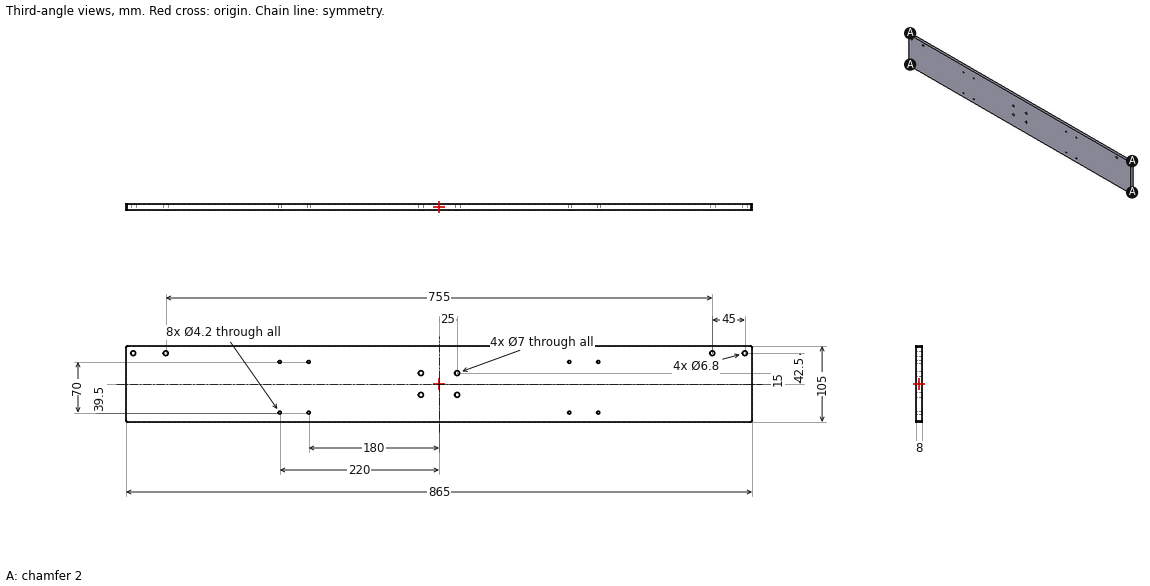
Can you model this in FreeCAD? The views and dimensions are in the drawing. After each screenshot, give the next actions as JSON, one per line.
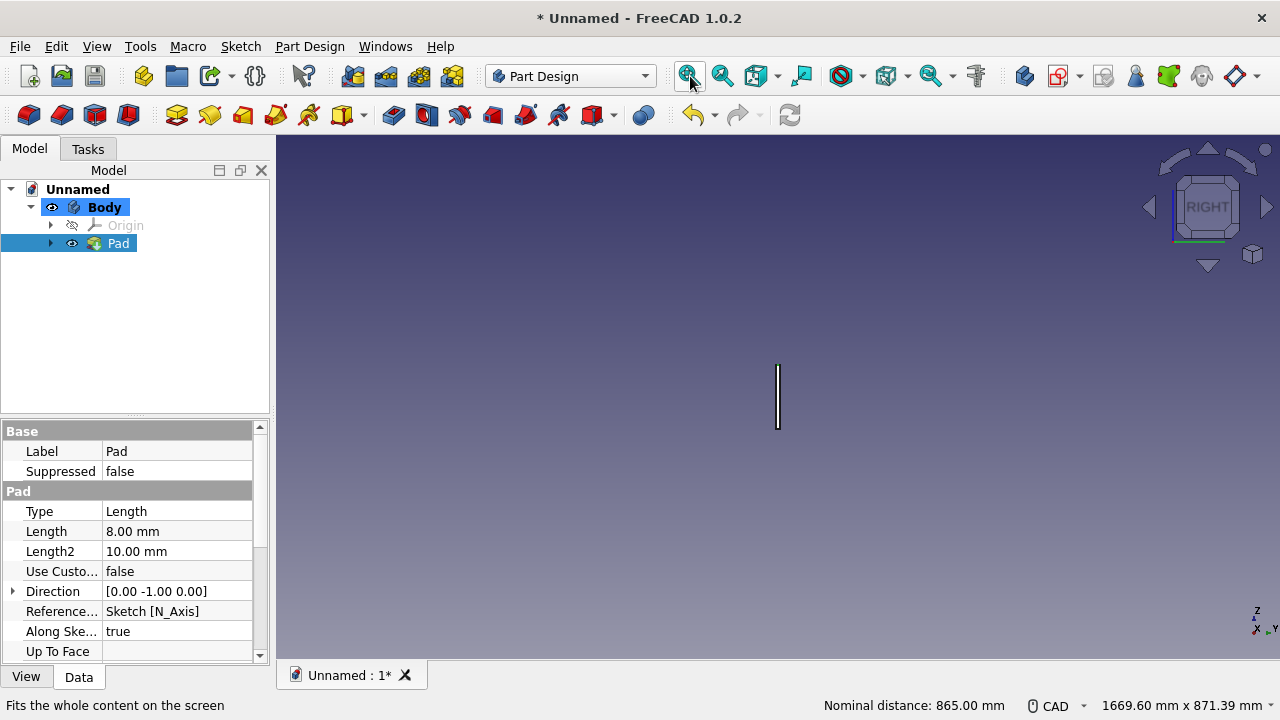
{"action": "scroll", "coordinate": [778, 428], "scroll_direction": "up", "scroll_amount": 11}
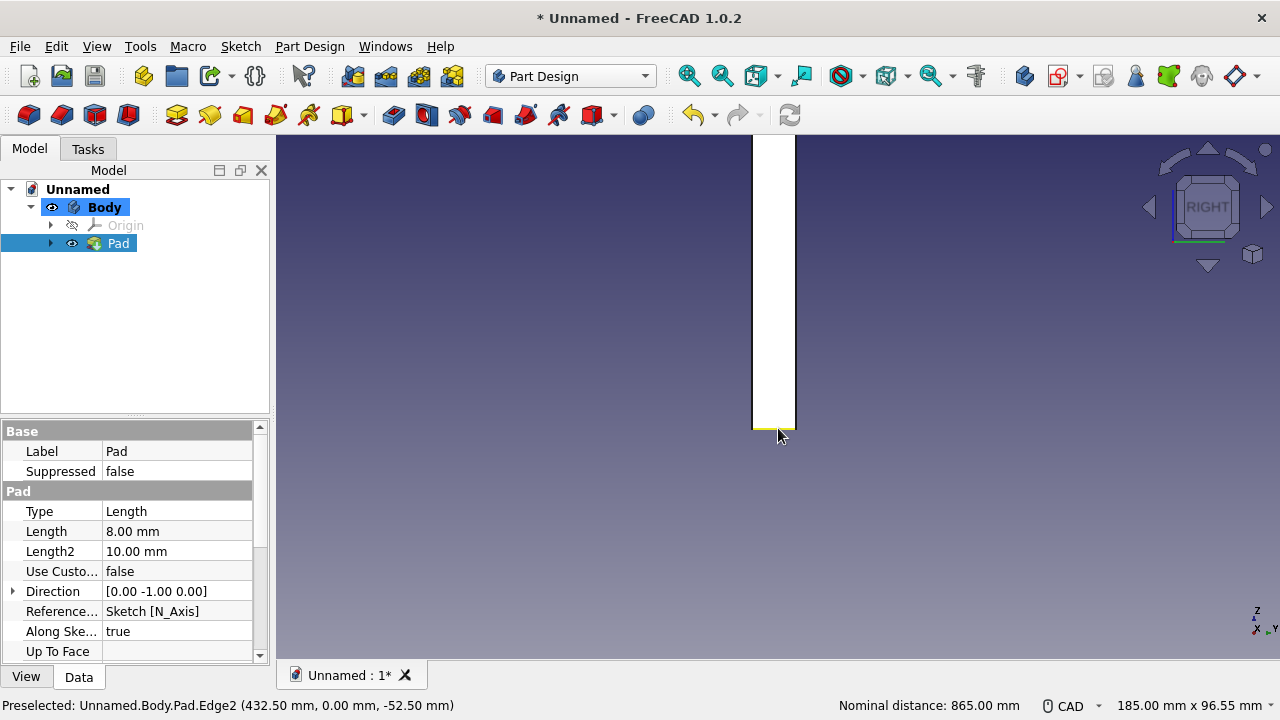
{"action": "left_click", "coordinate": [774, 428], "text": "ctrl"}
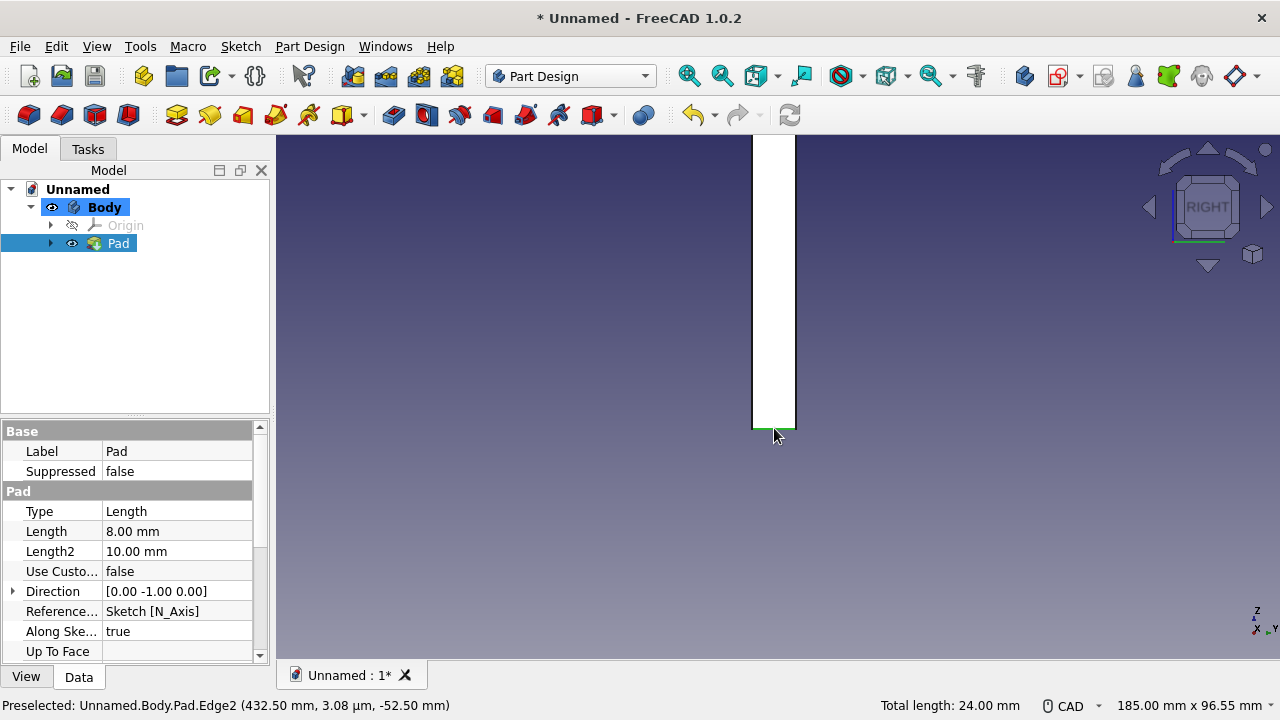
{"action": "key", "text": "v f"}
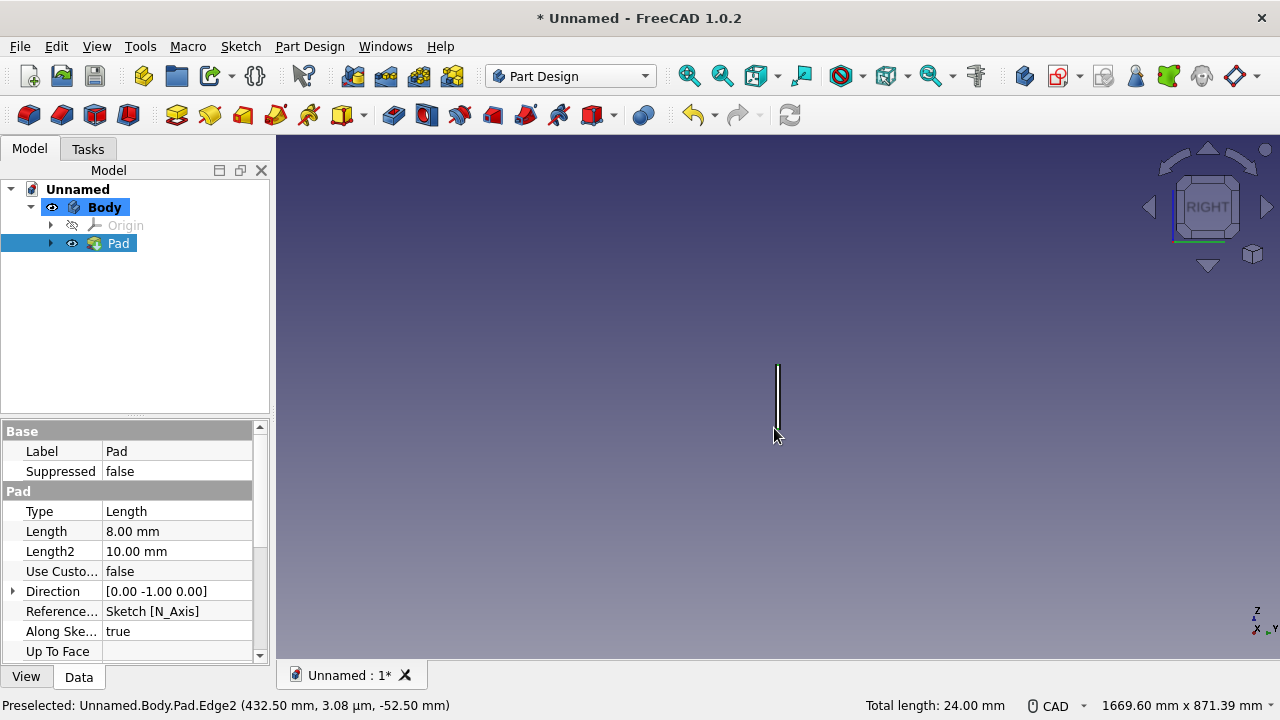
{"action": "key", "text": "5"}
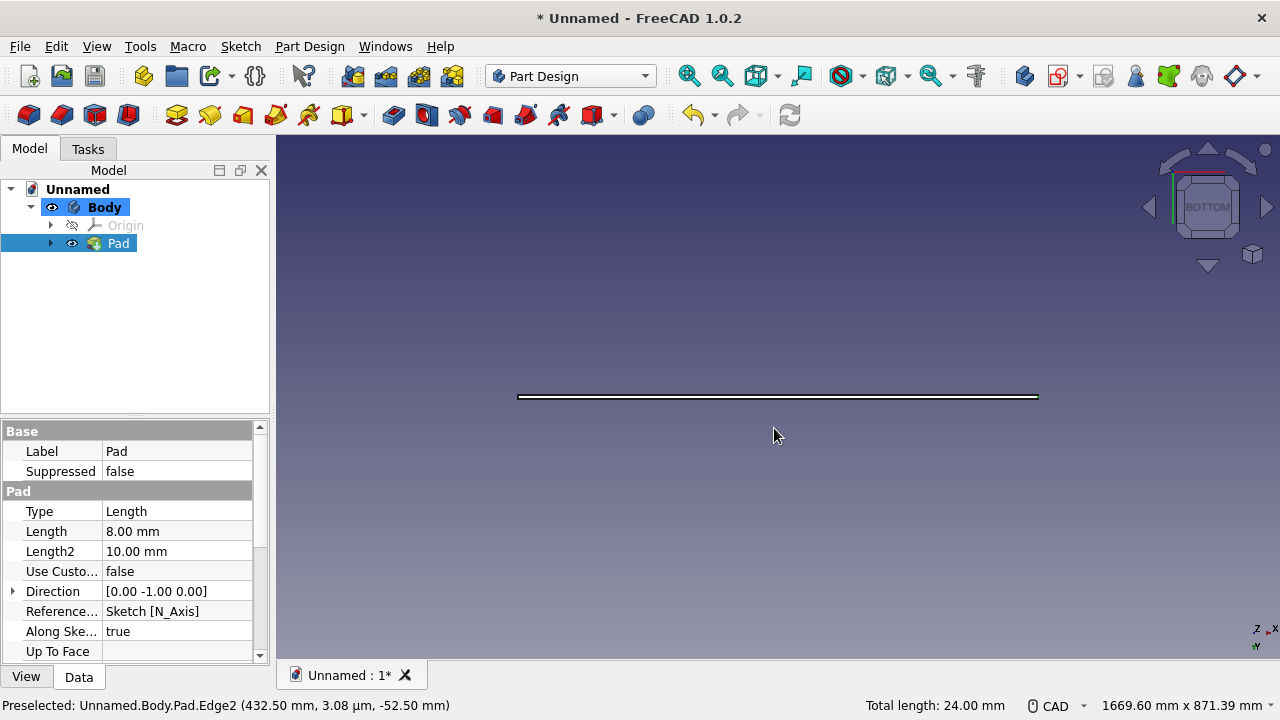
{"action": "scroll", "coordinate": [518, 396], "scroll_direction": "up", "scroll_amount": 11}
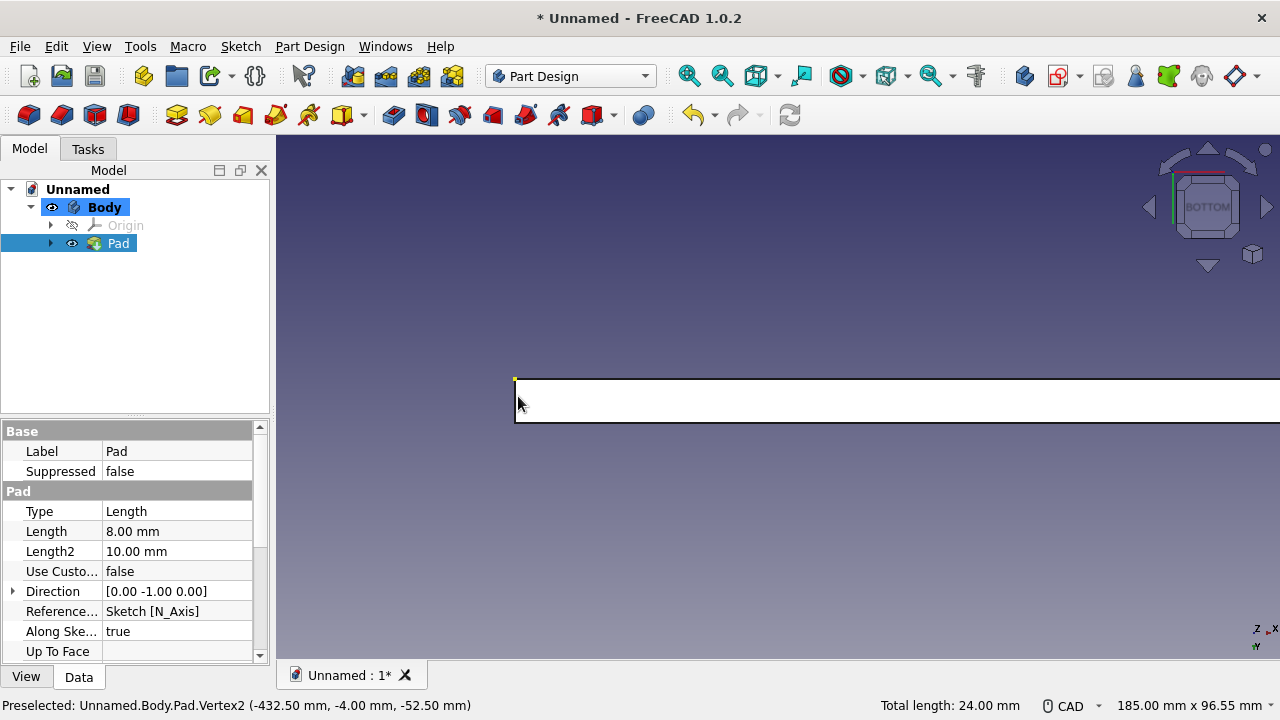
{"action": "left_click", "coordinate": [515, 400], "text": "ctrl"}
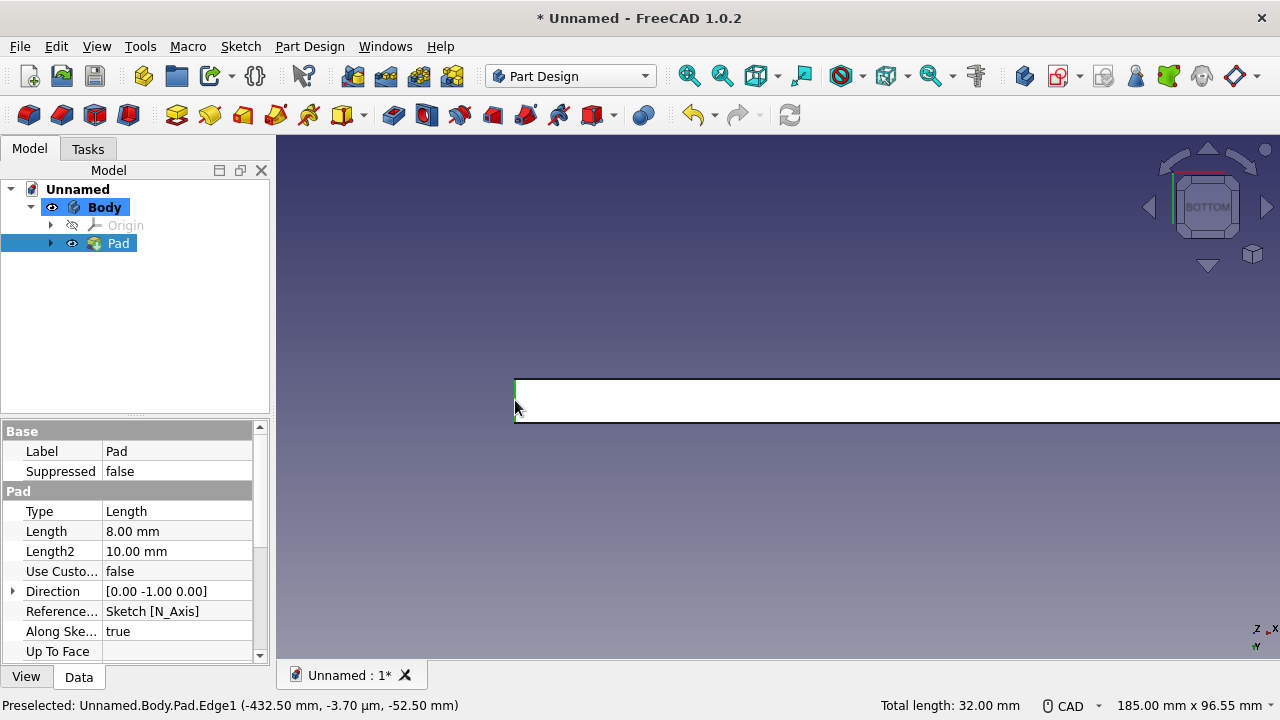
{"action": "left_click", "coordinate": [62, 116]}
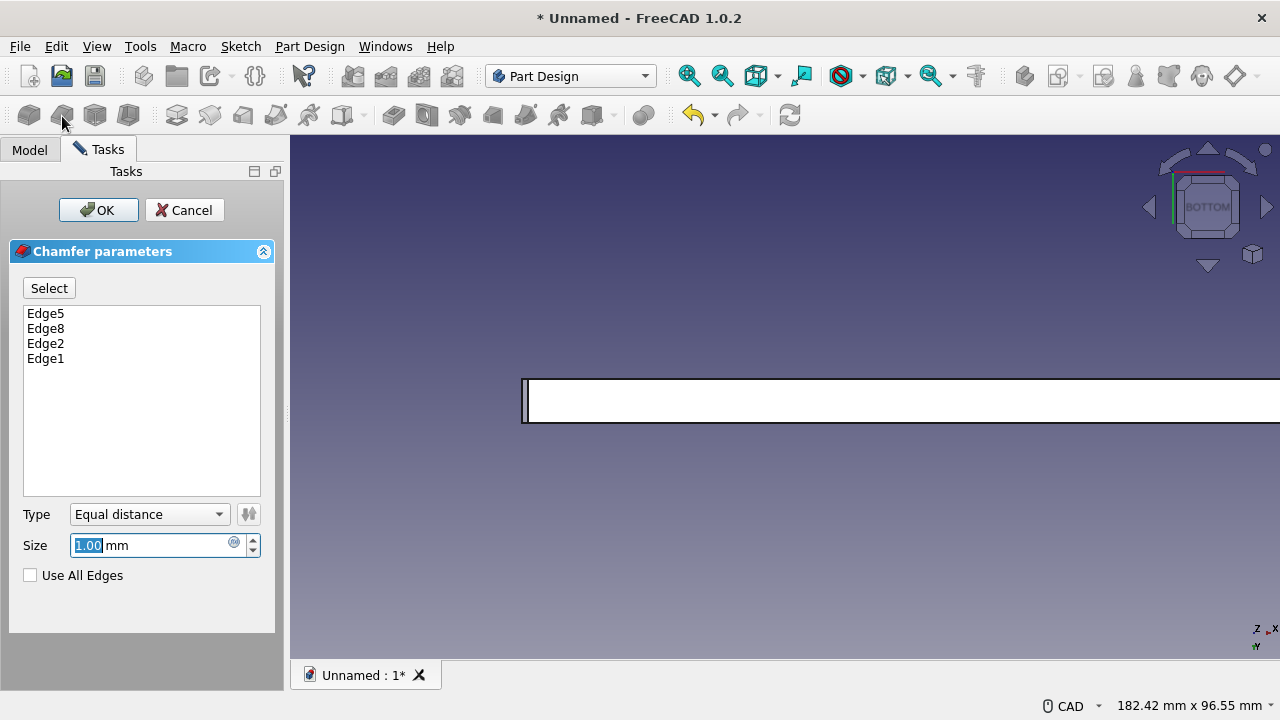
{"action": "type", "text": "2"}
{"action": "key", "text": "Tab"}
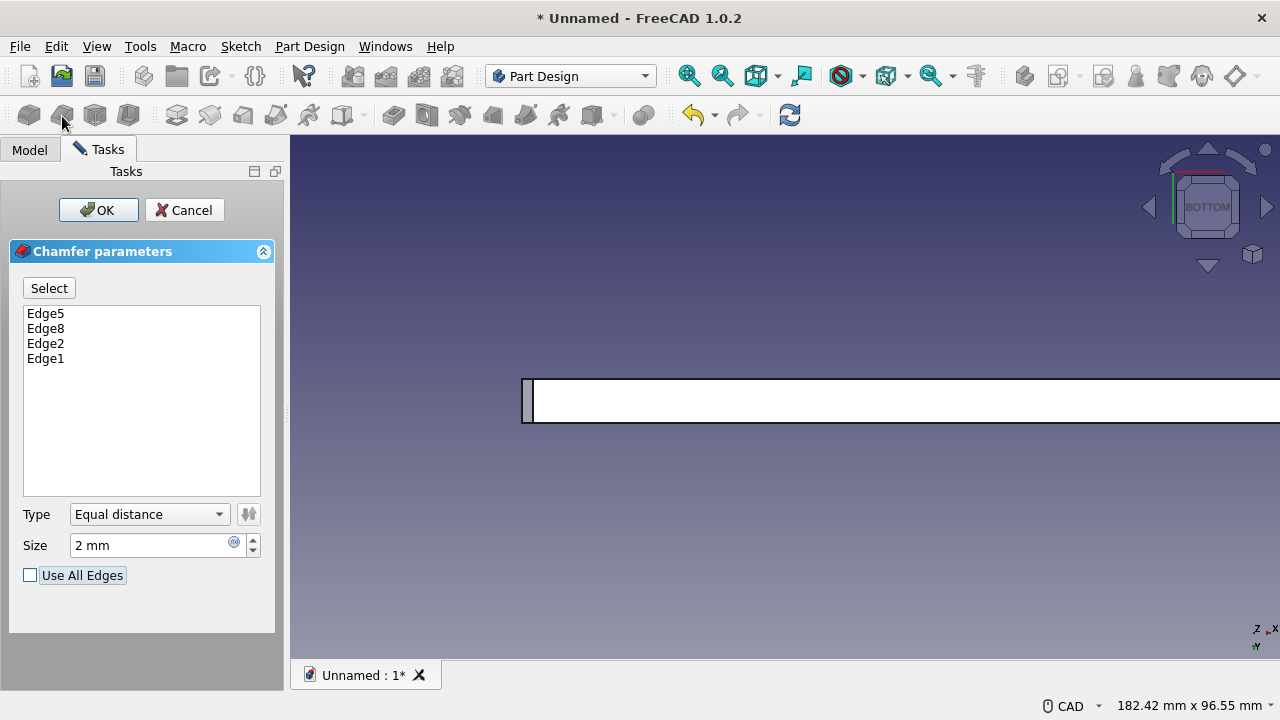
{"action": "left_click", "coordinate": [99, 210]}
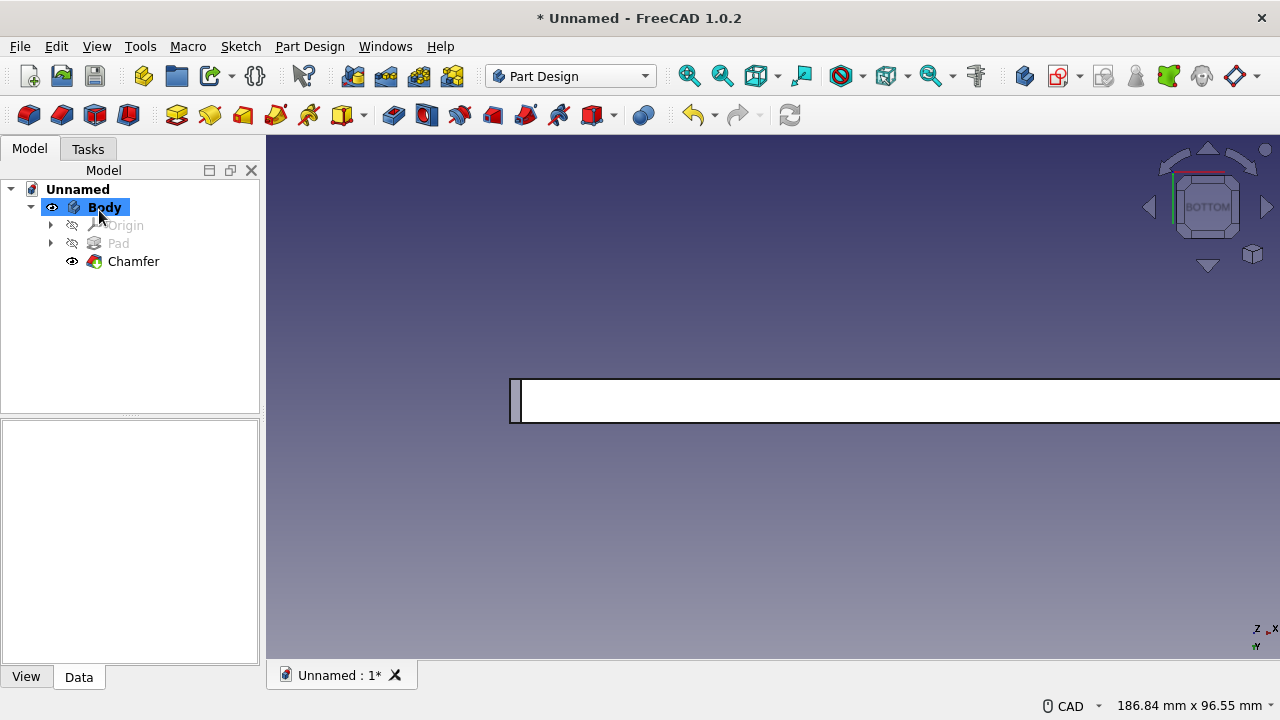
{"action": "left_click", "coordinate": [690, 76]}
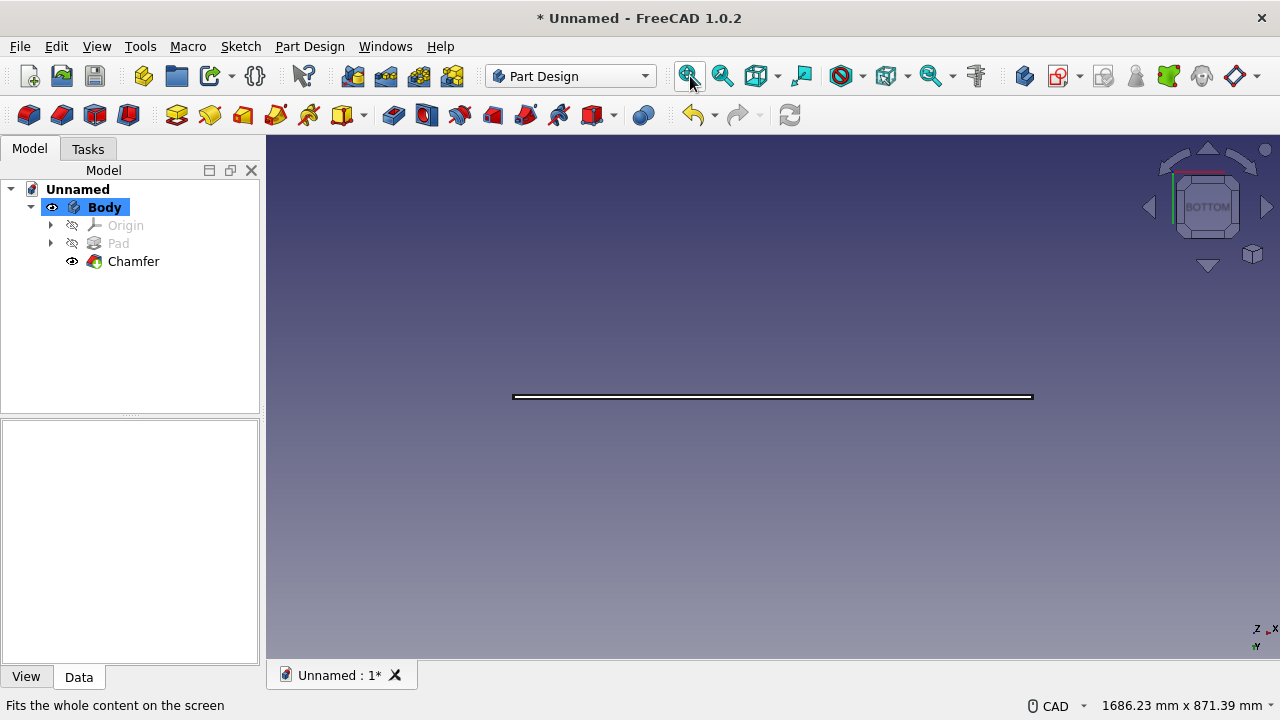
{"action": "key", "text": "4"}